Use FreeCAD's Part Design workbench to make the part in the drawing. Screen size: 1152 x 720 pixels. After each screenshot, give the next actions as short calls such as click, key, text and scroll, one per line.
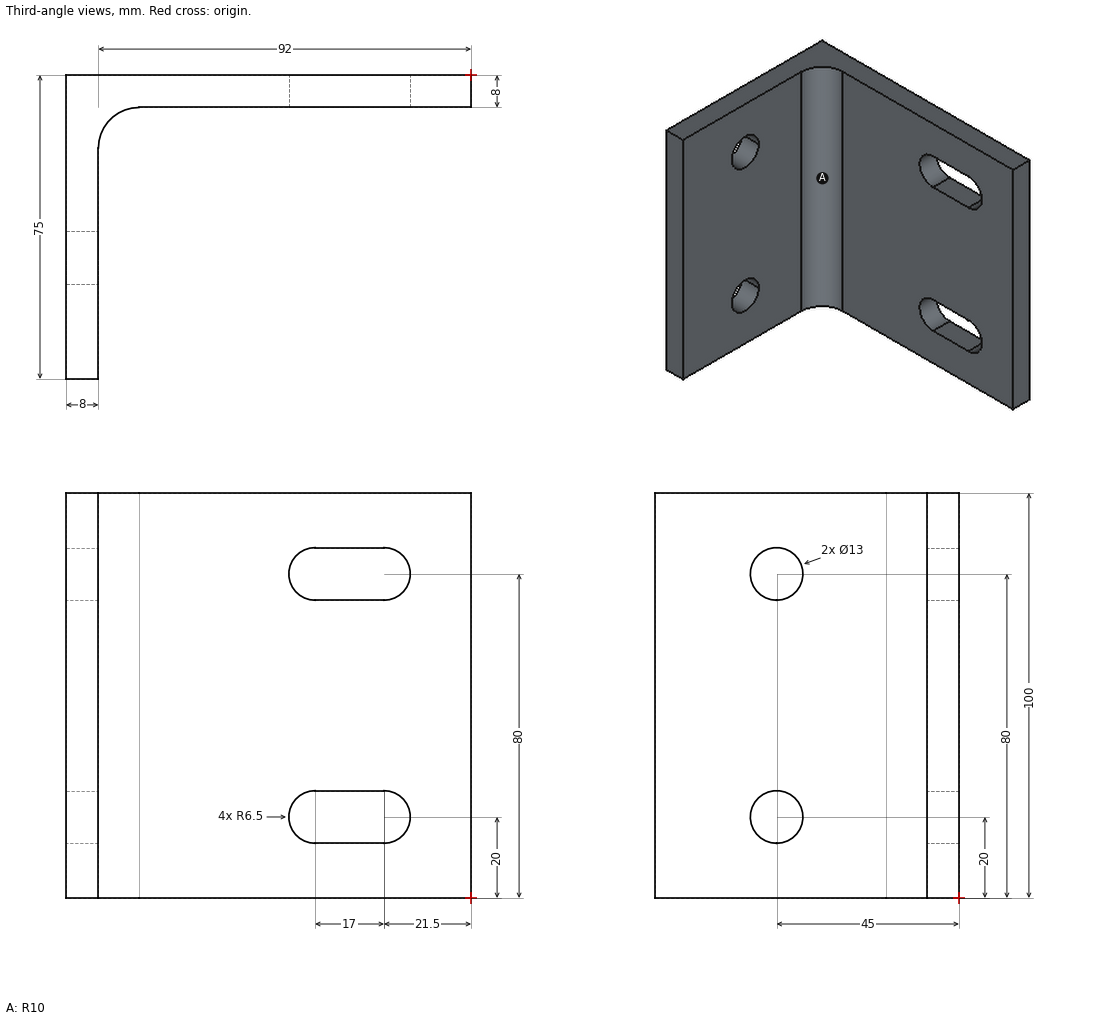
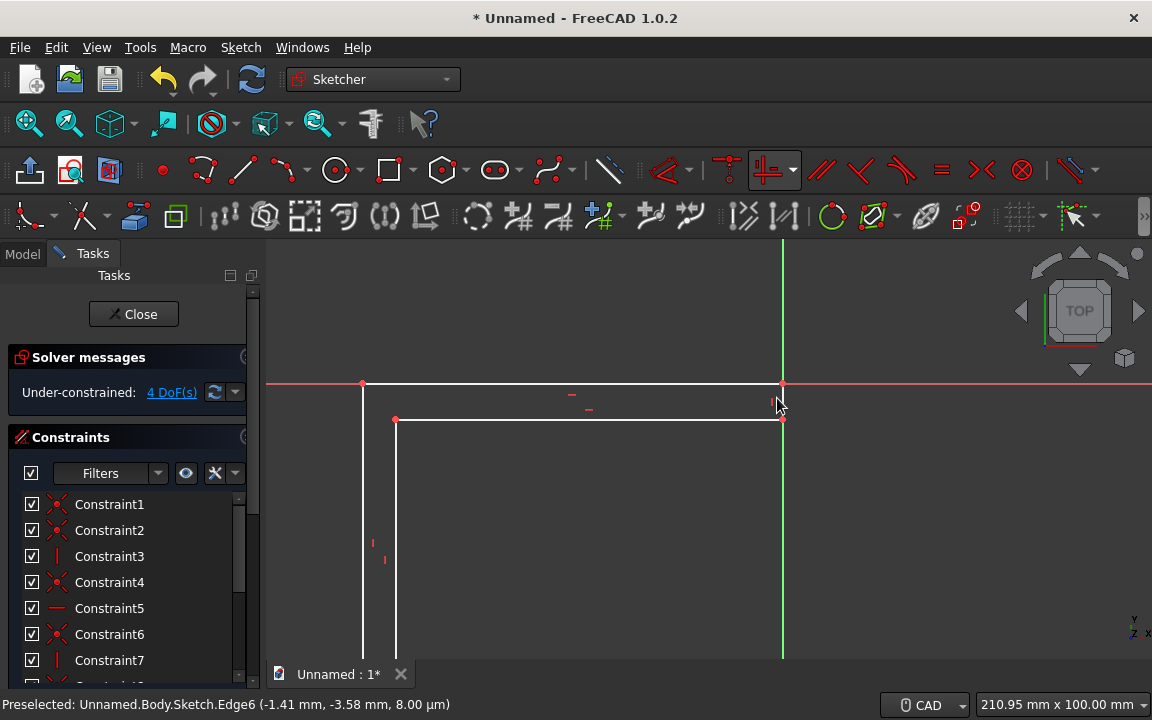
click(664, 170)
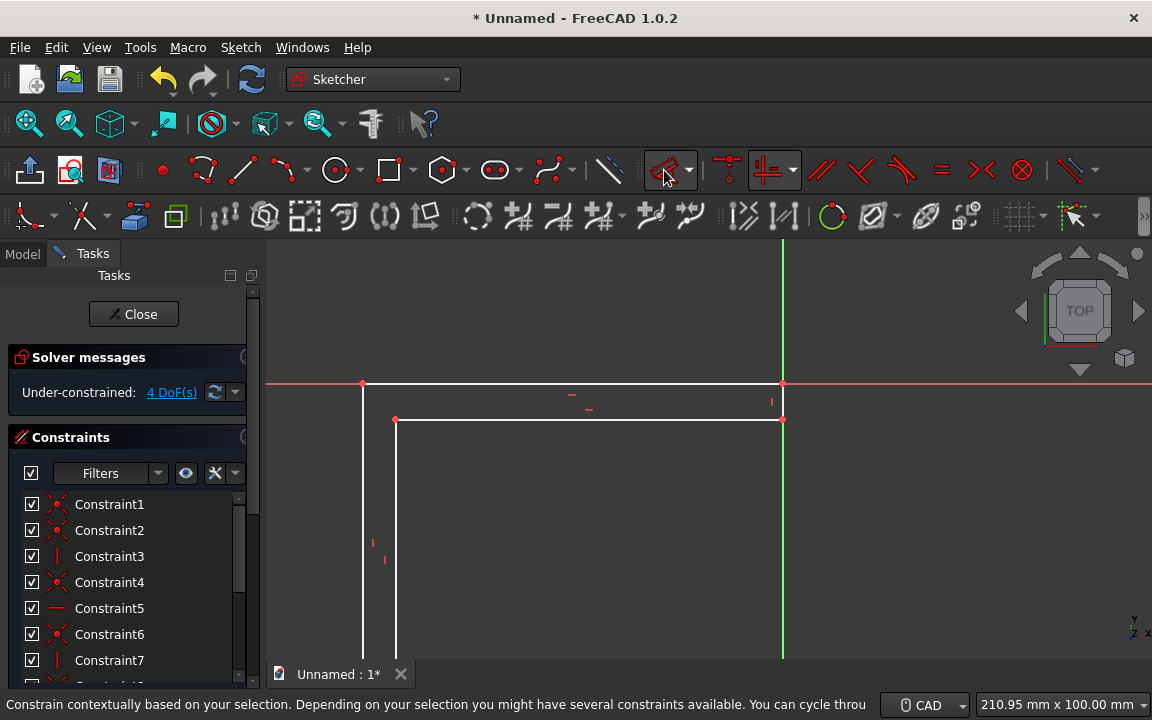
scroll(778, 267, down, 2)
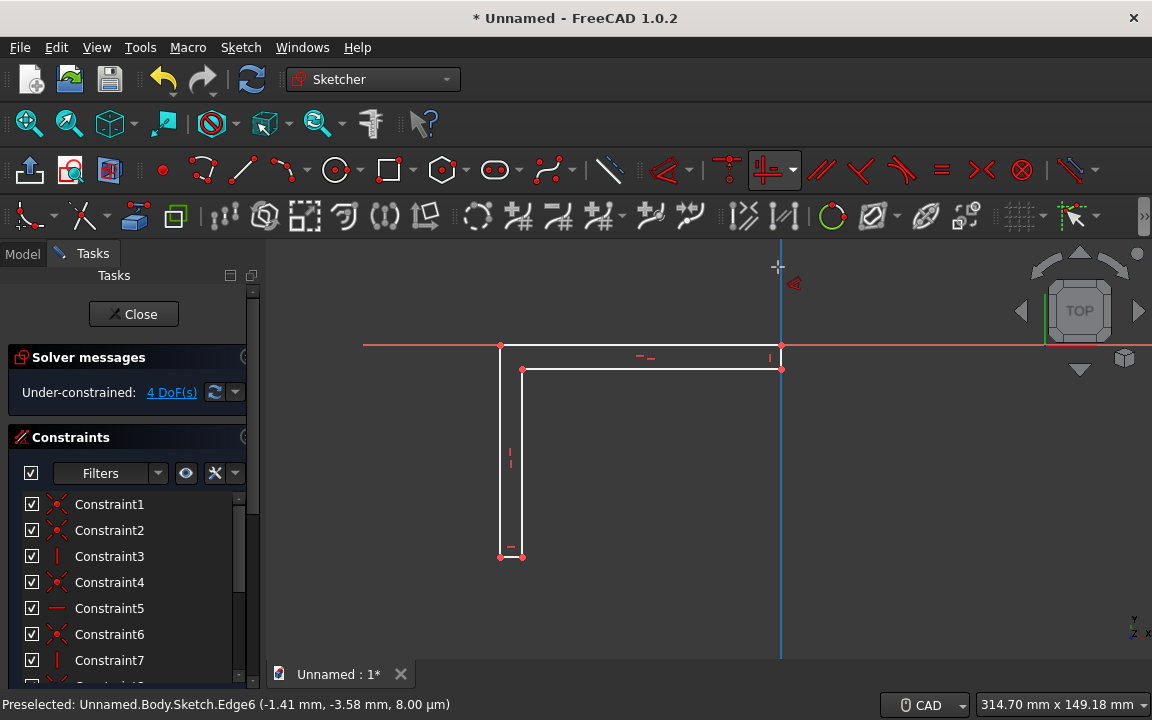
scroll(507, 557, up, 4)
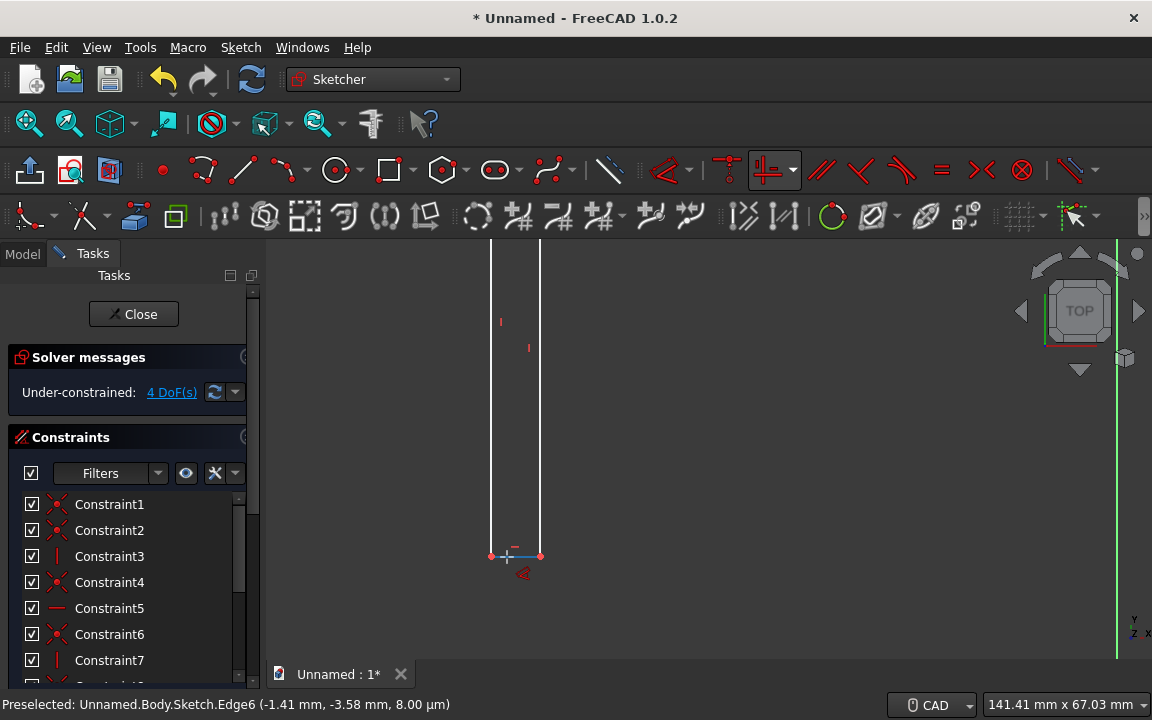
click(506, 557)
click(516, 591)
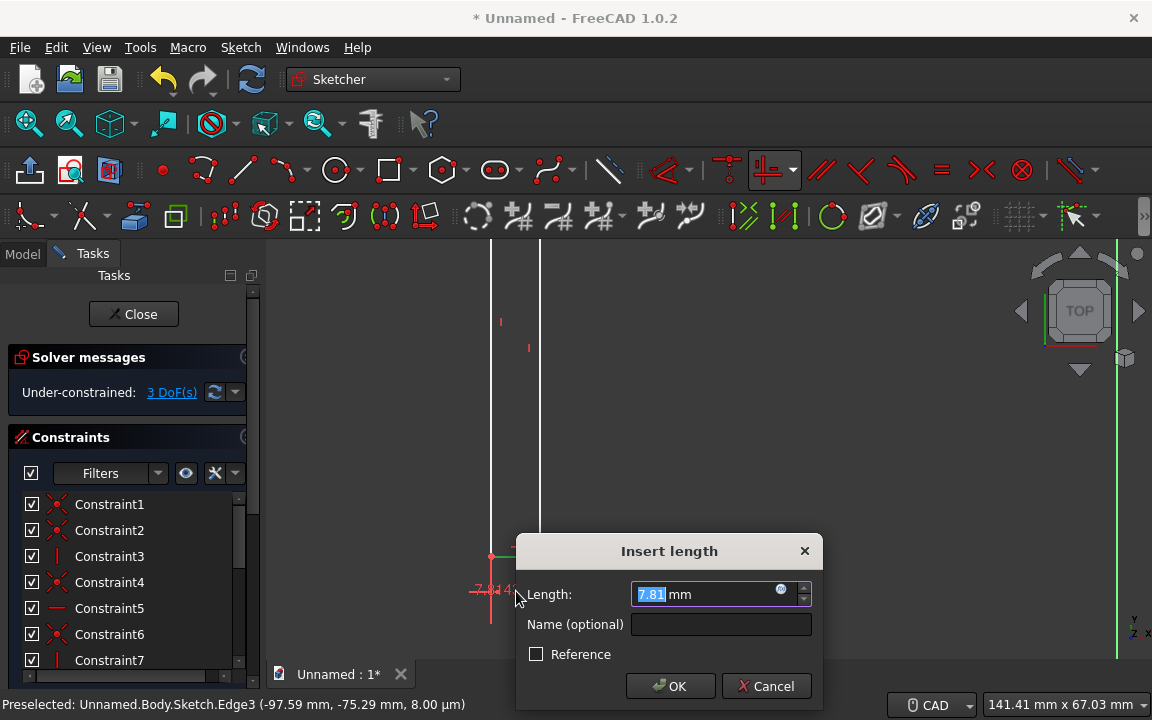
text(8)
key(Return)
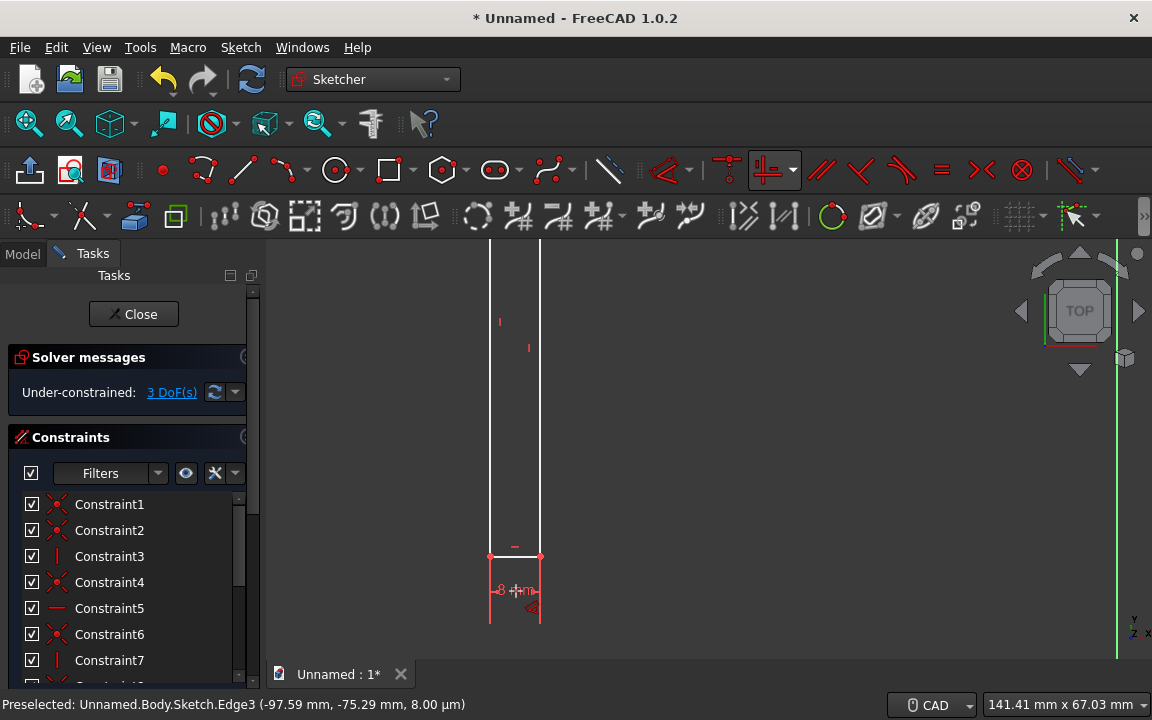
scroll(441, 606, down, 3)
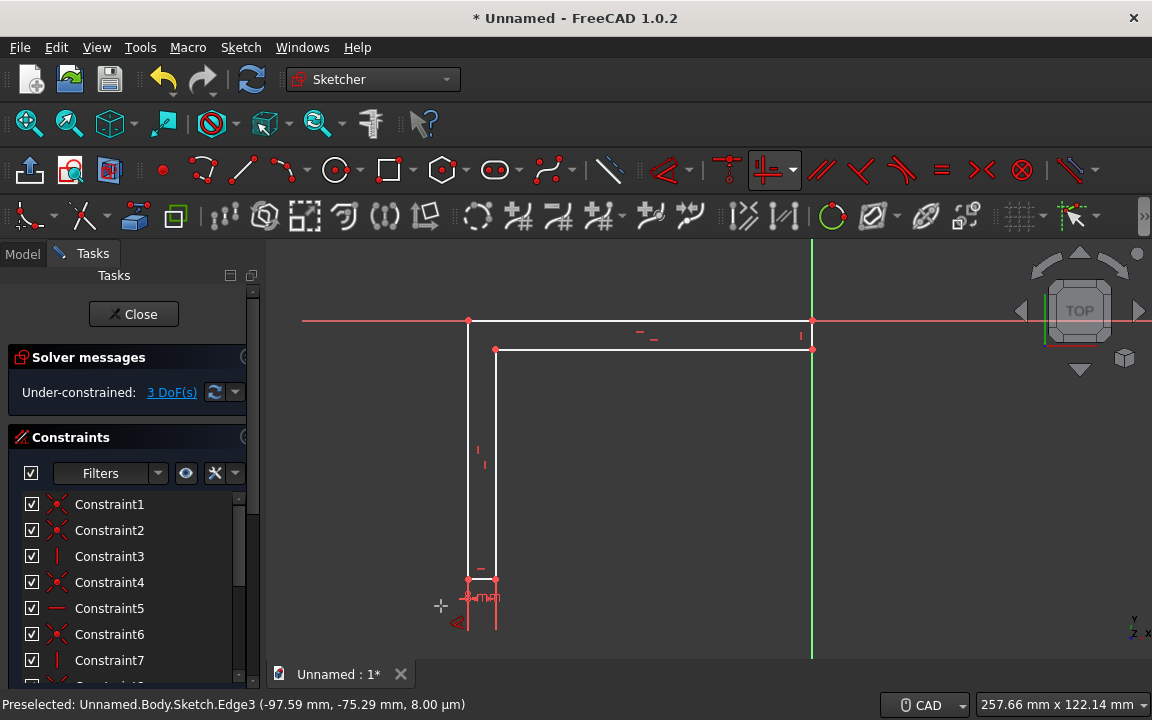
scroll(812, 341, up, 3)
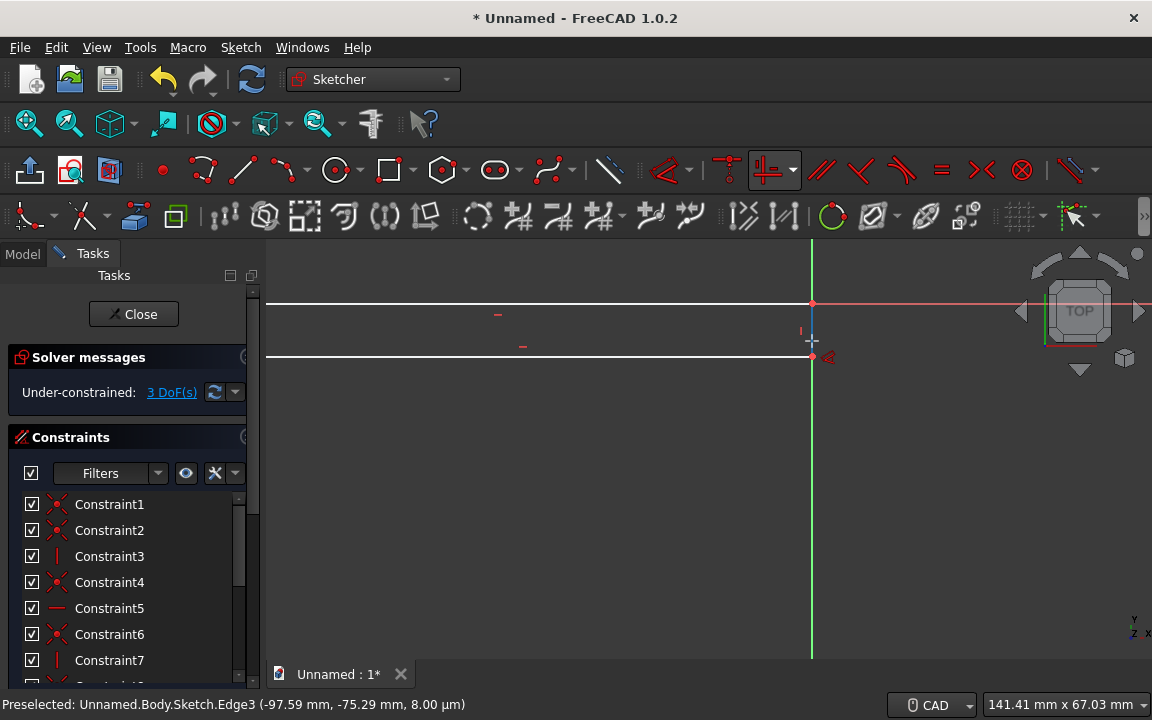
click(812, 341)
click(846, 330)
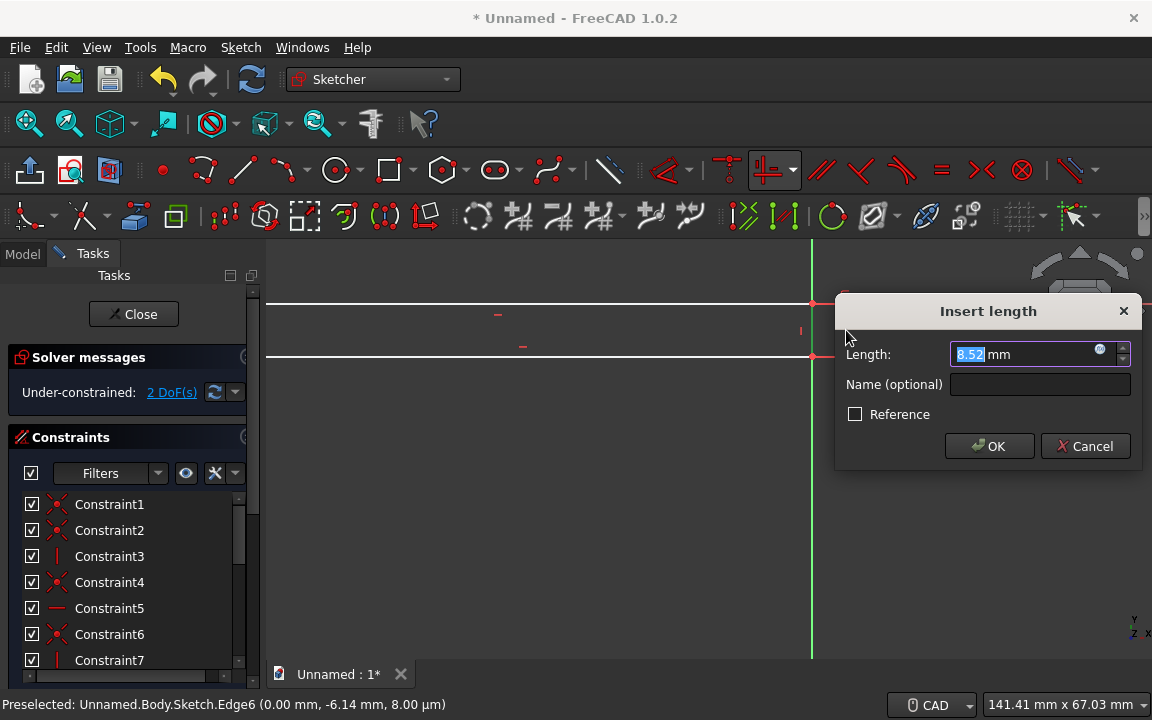
text(8)
key(Return)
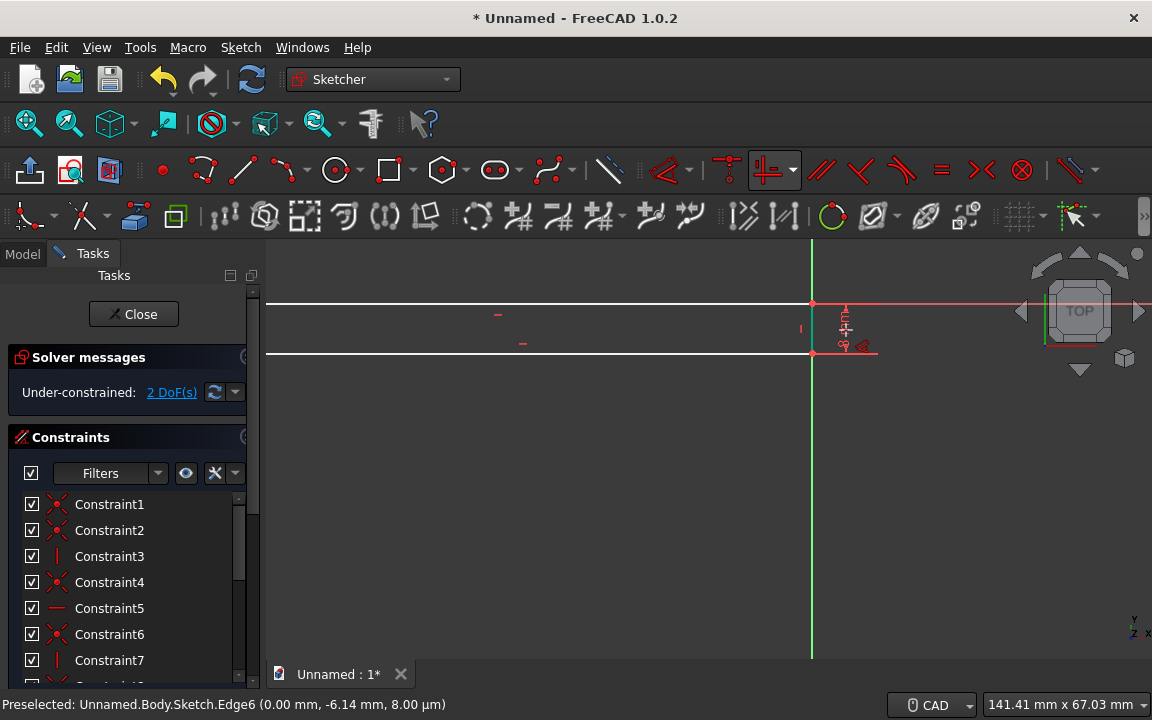
scroll(813, 340, down, 3)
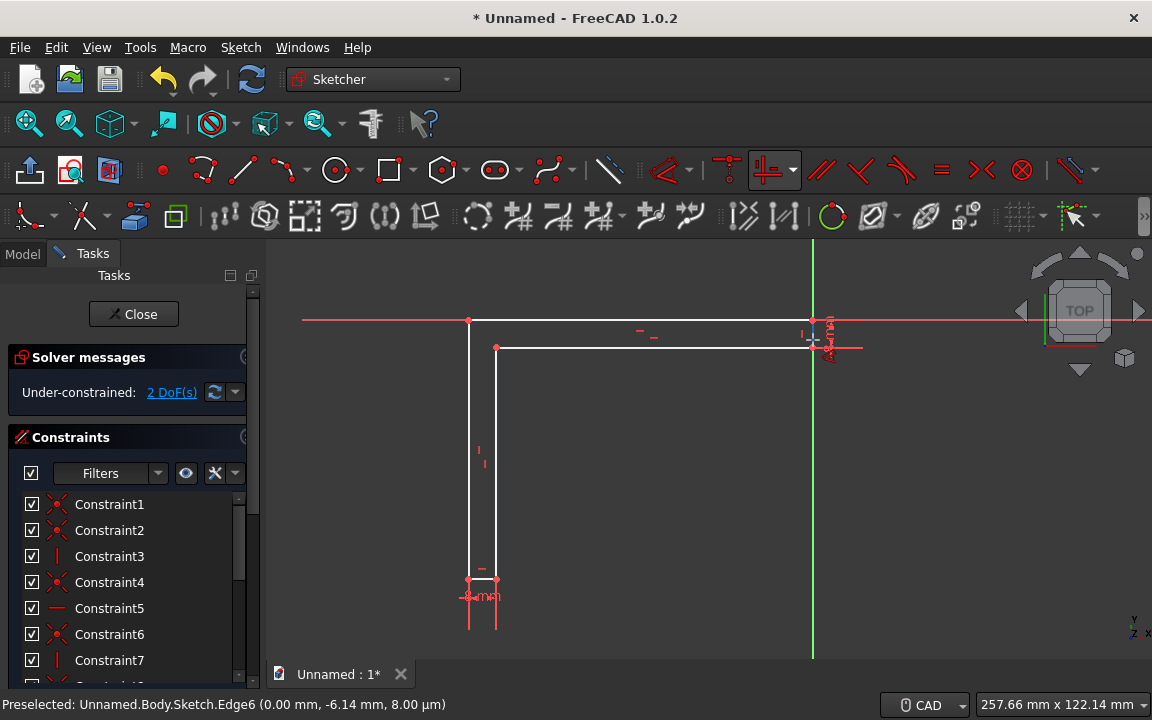
click(469, 398)
click(435, 450)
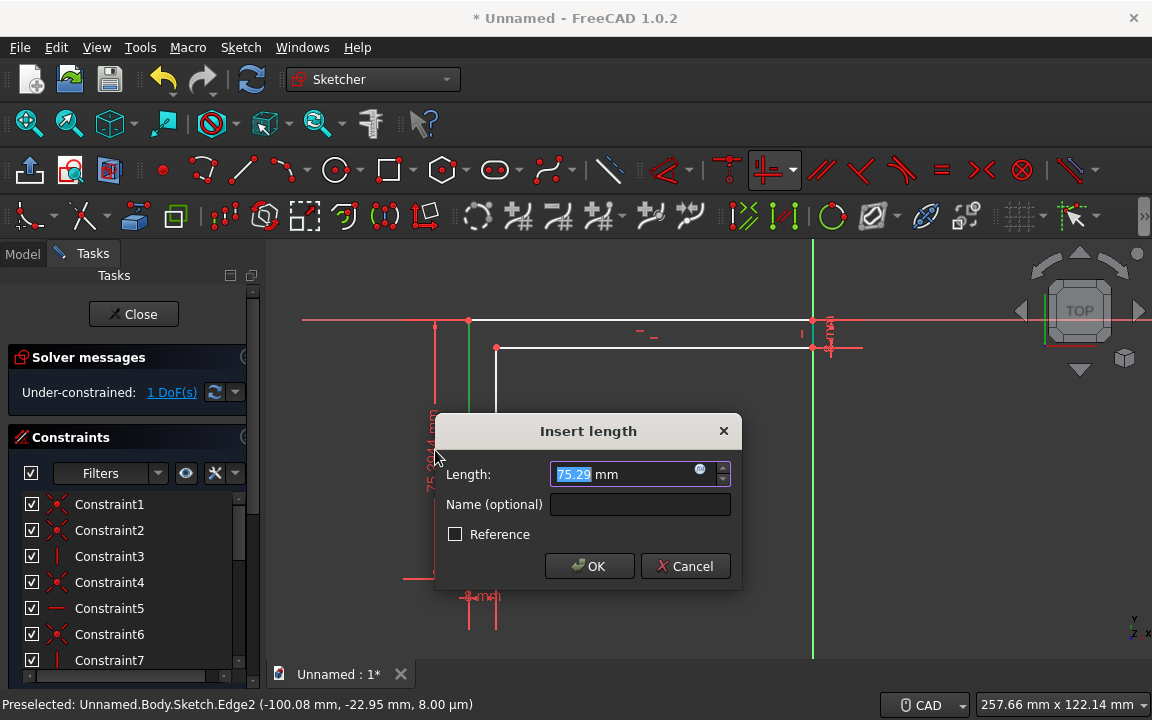
text(75)
key(Return)